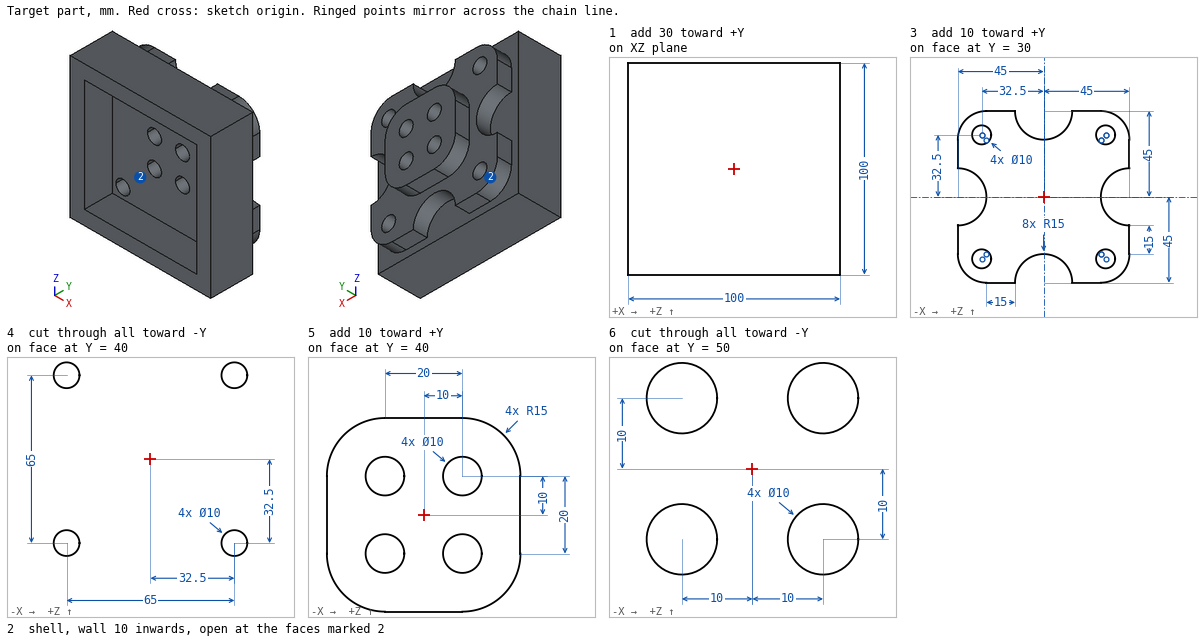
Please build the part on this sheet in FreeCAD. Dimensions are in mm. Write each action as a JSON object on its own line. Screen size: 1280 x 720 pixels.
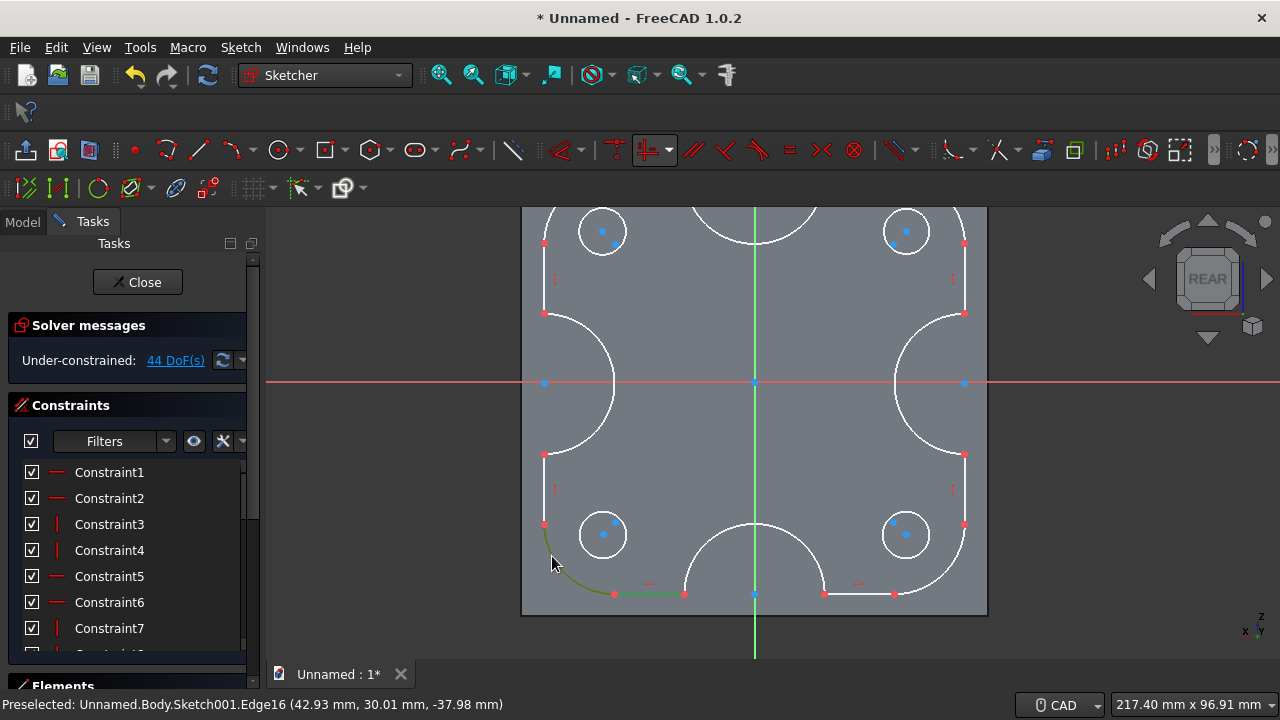
{"action": "left_click", "coordinate": [758, 150]}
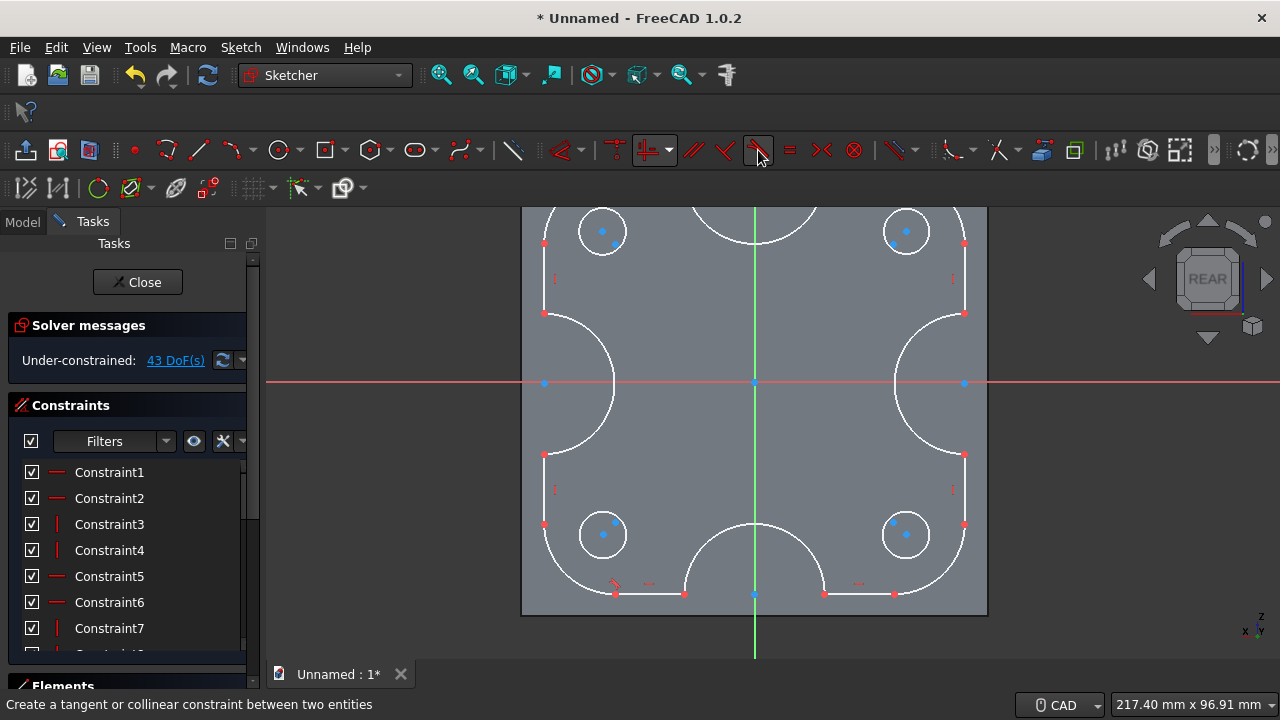
{"action": "left_click", "coordinate": [846, 594]}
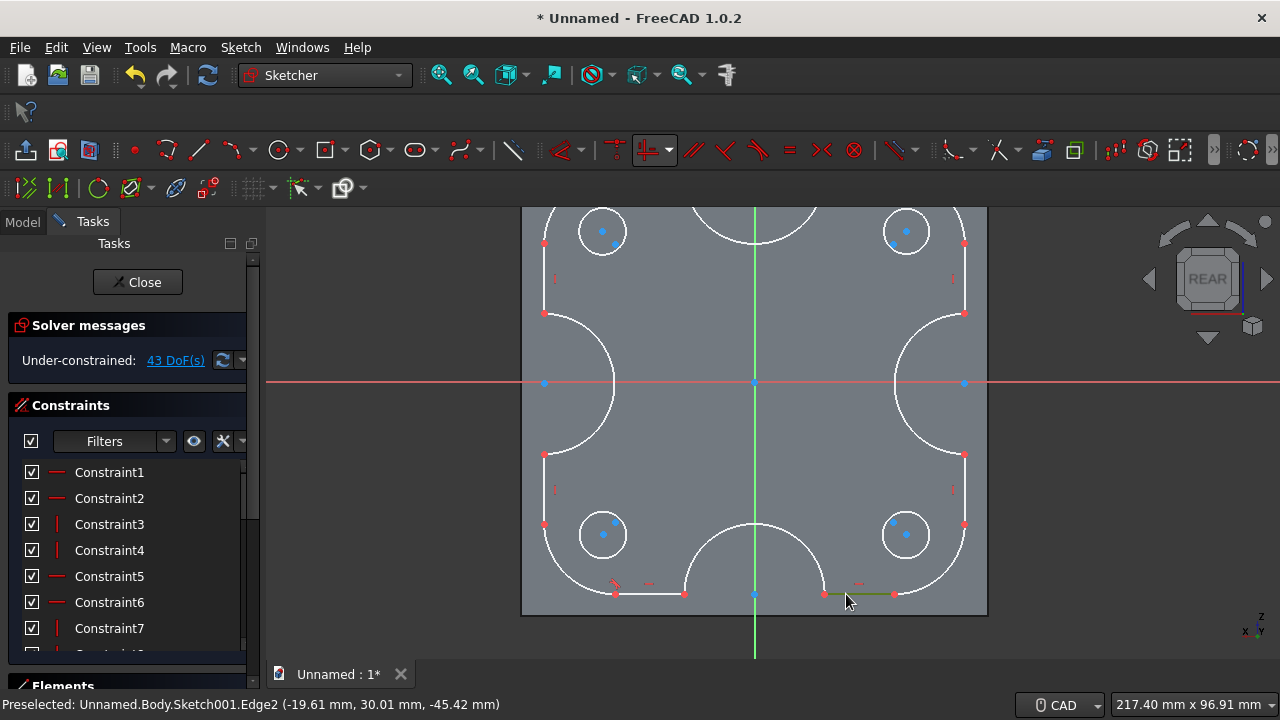
{"action": "left_click", "coordinate": [926, 586]}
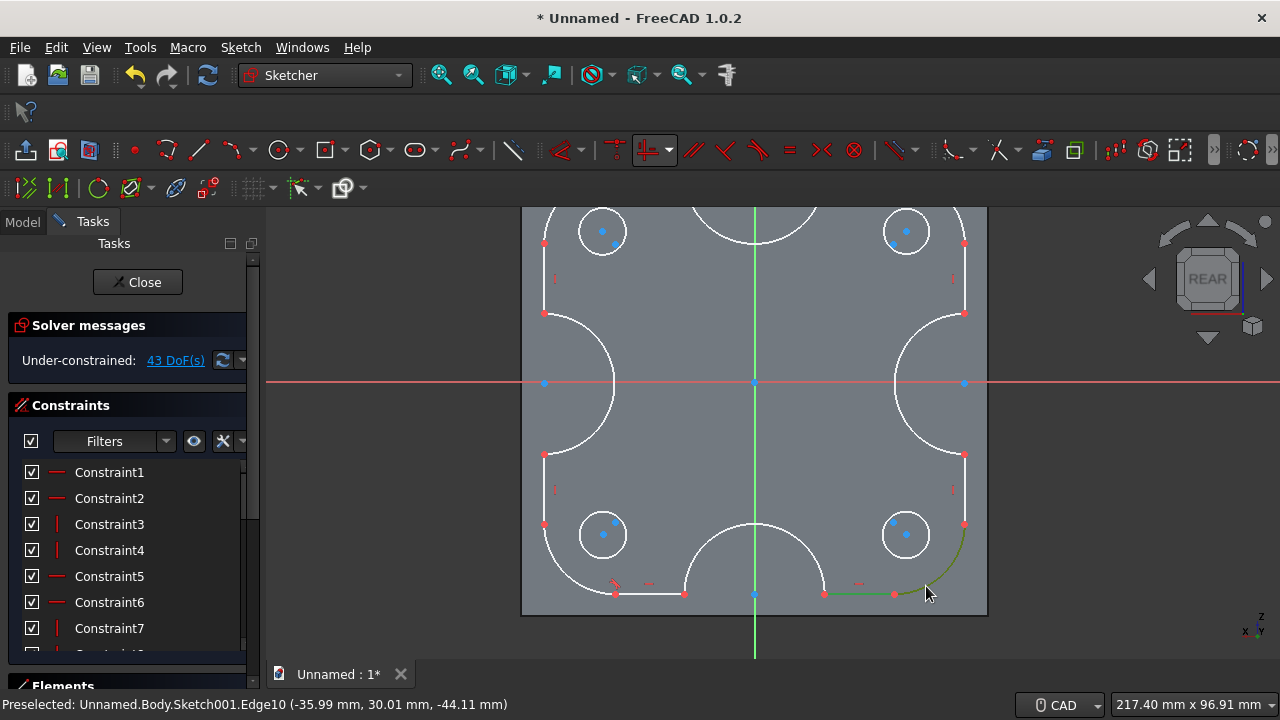
{"action": "left_click", "coordinate": [758, 150]}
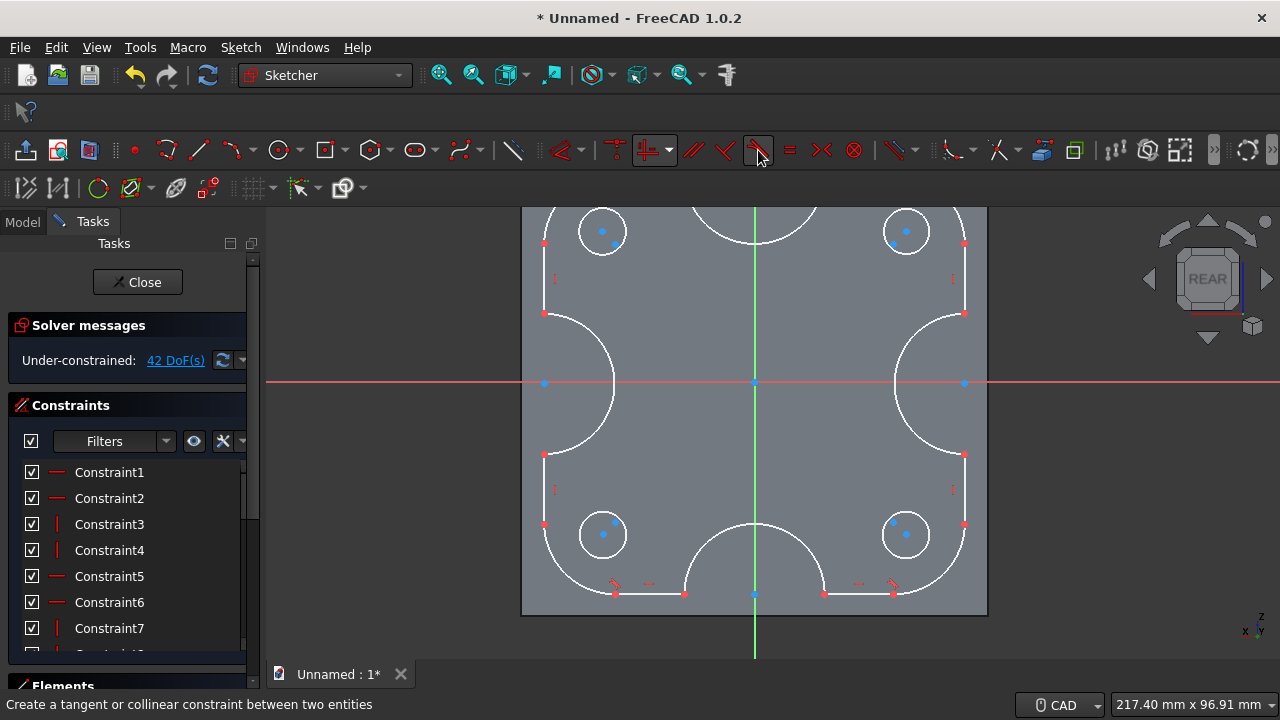
{"action": "left_click", "coordinate": [965, 503]}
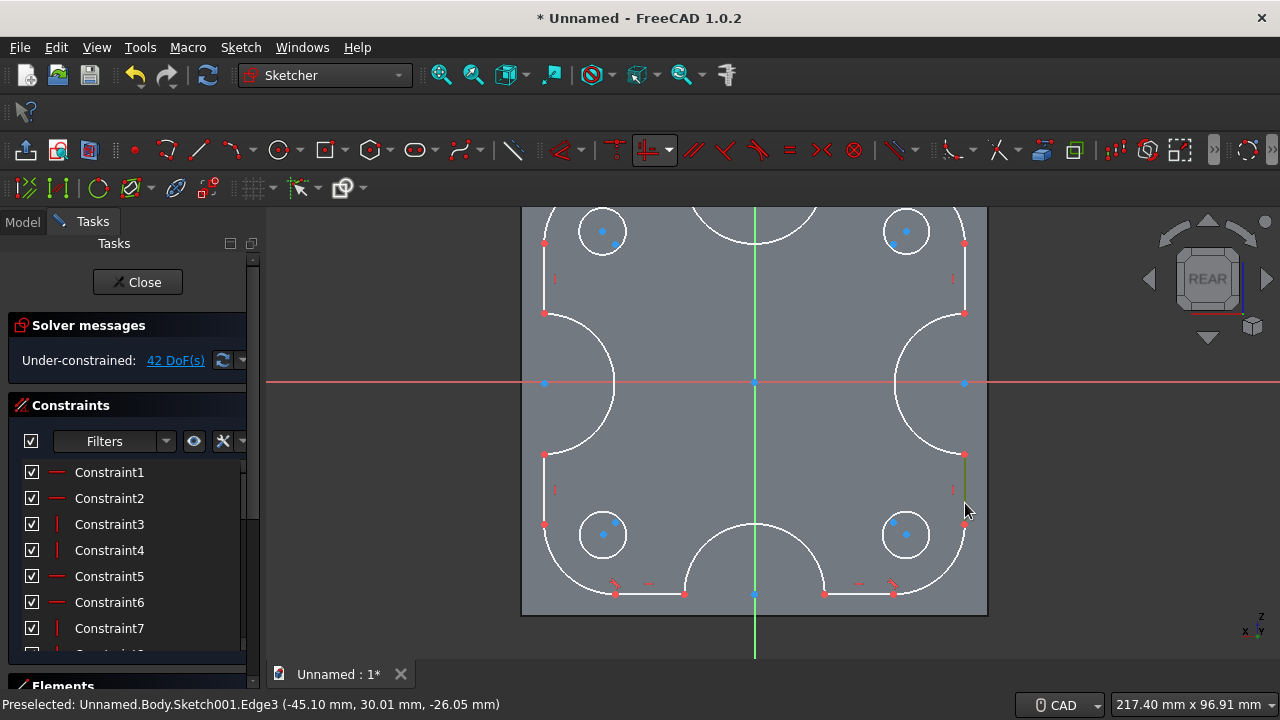
{"action": "left_click", "coordinate": [926, 587]}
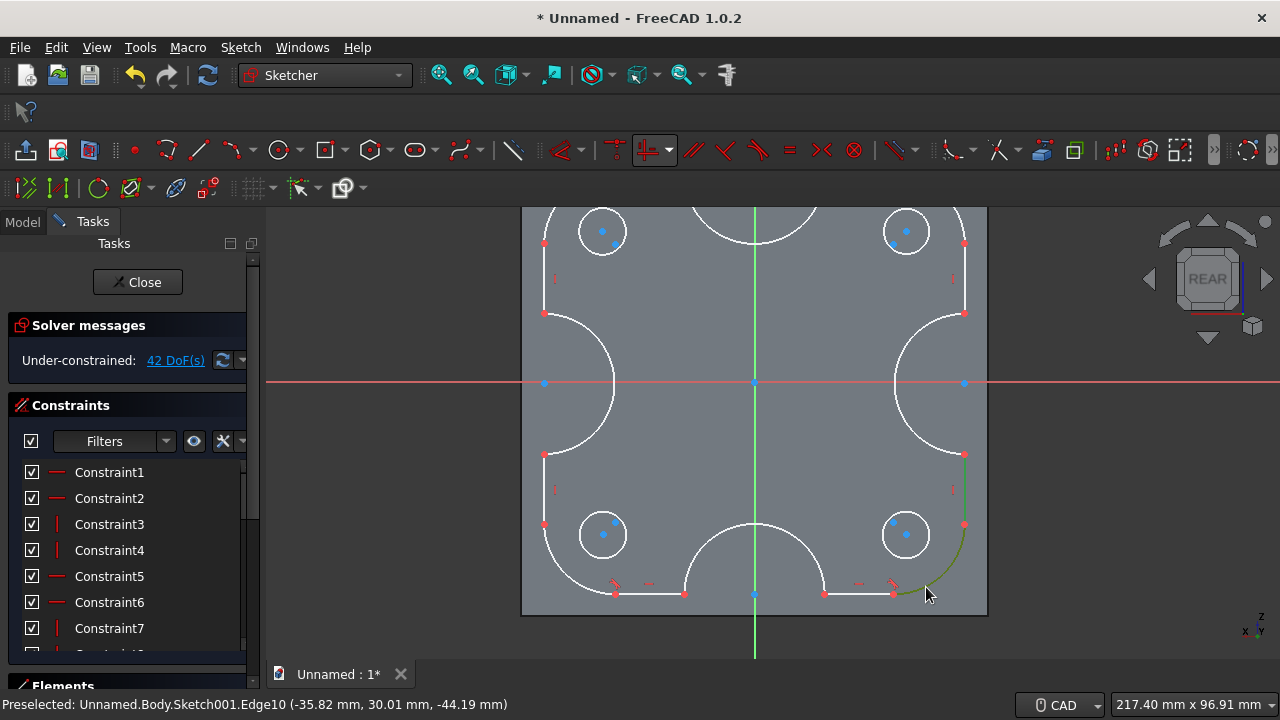
{"action": "left_click", "coordinate": [758, 150]}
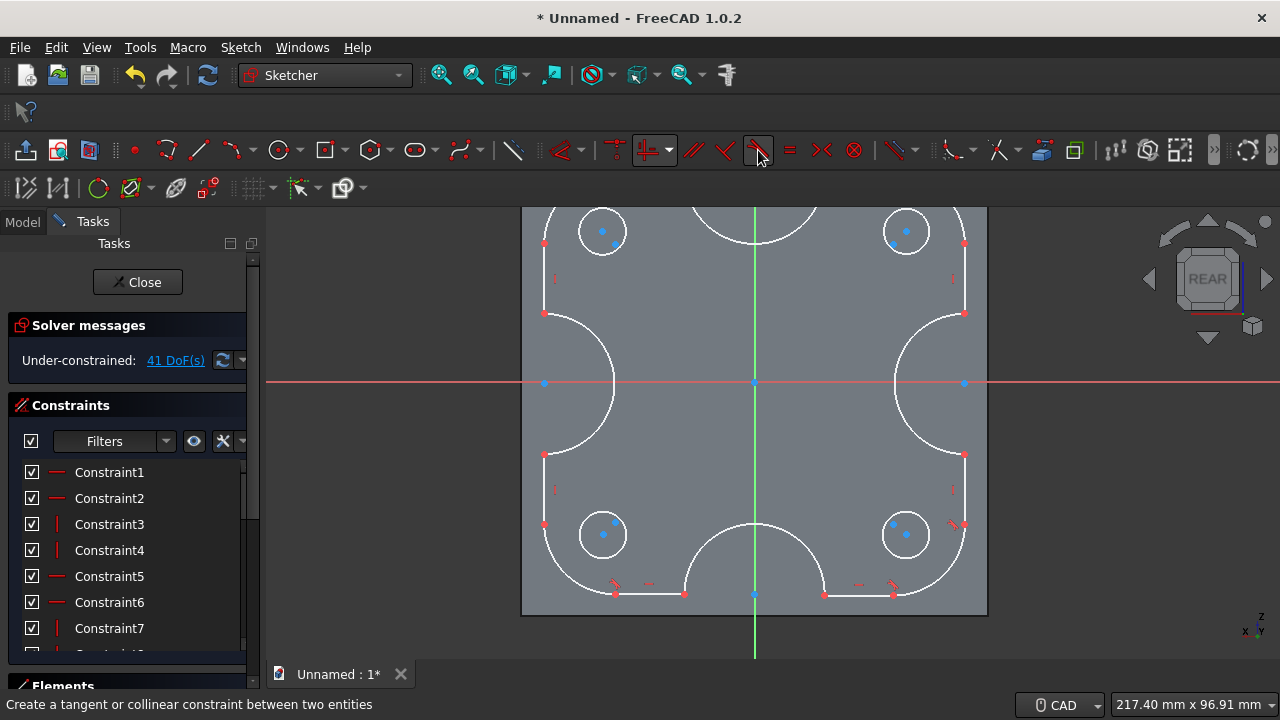
{"action": "left_click", "coordinate": [965, 293]}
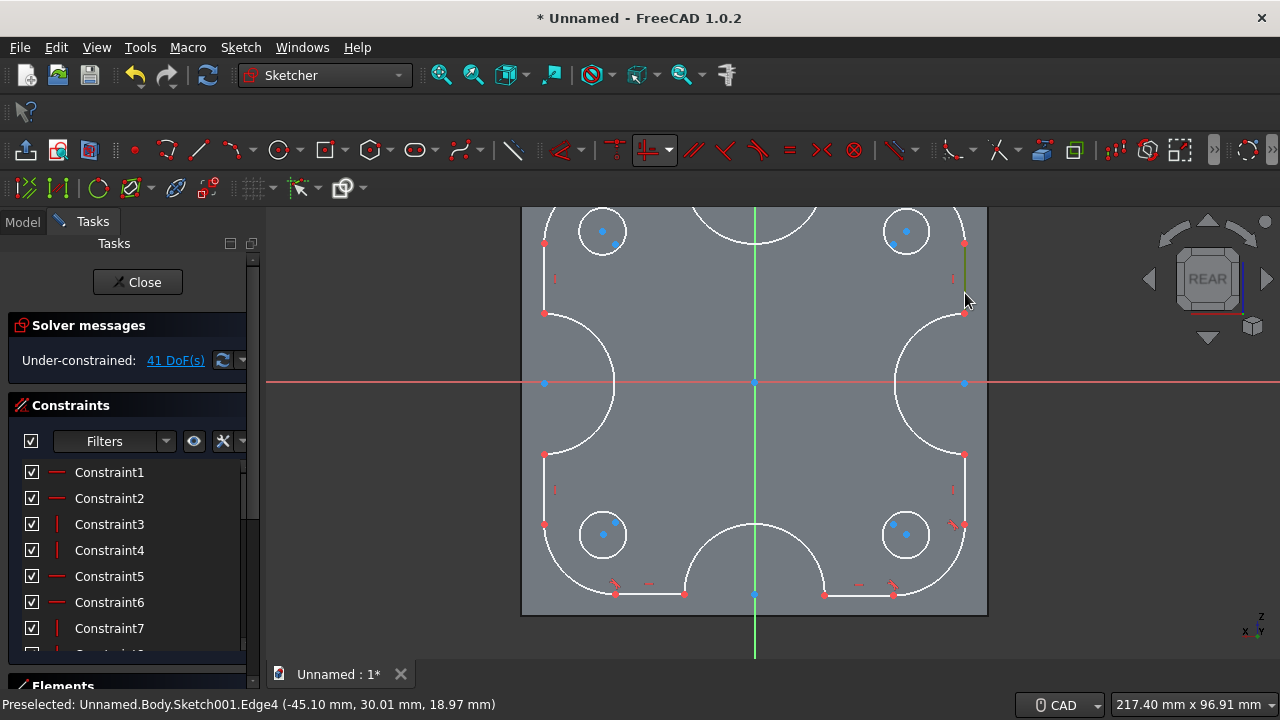
{"action": "scroll", "coordinate": [603, 536], "scroll_direction": "down", "scroll_amount": 2}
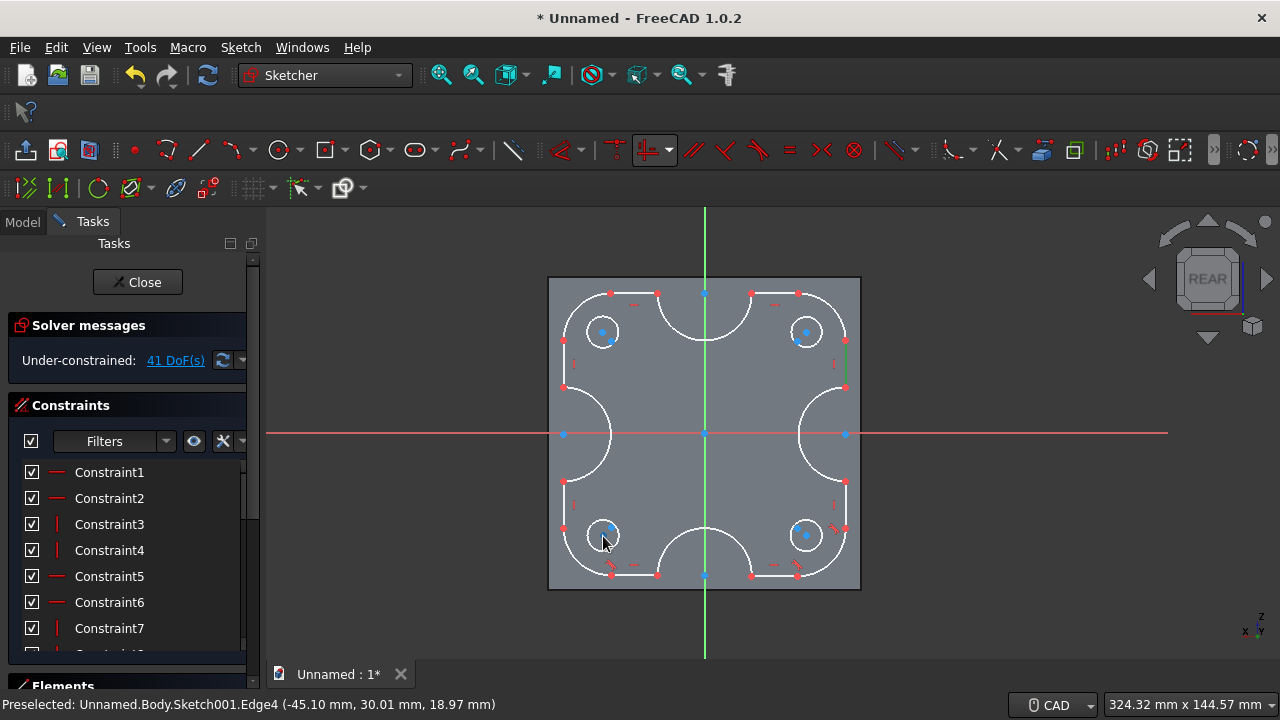
{"action": "left_click", "coordinate": [840, 319]}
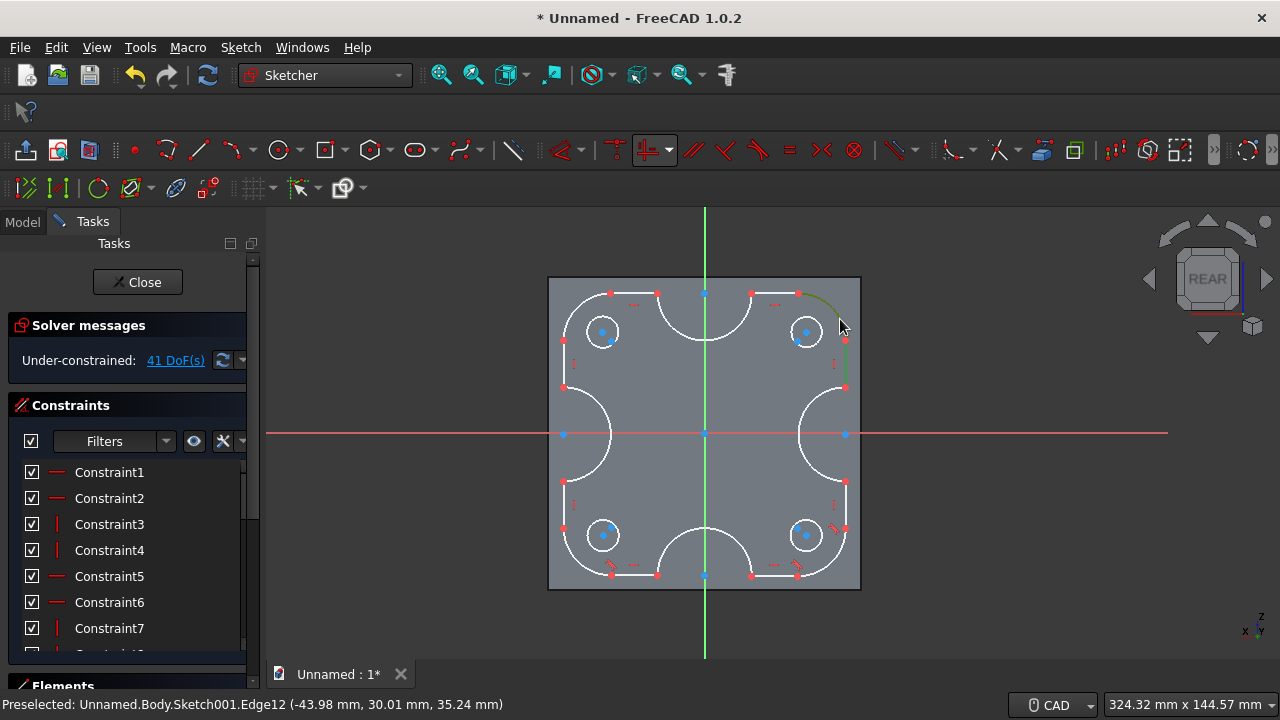
{"action": "left_click", "coordinate": [758, 150]}